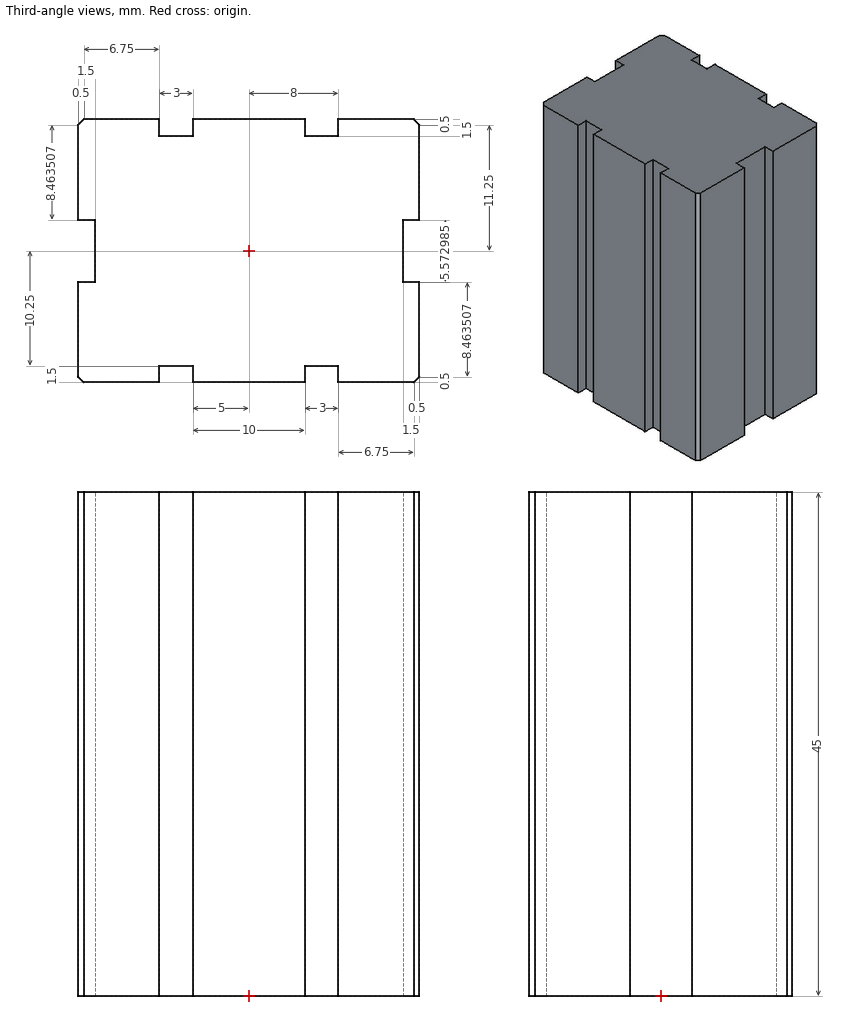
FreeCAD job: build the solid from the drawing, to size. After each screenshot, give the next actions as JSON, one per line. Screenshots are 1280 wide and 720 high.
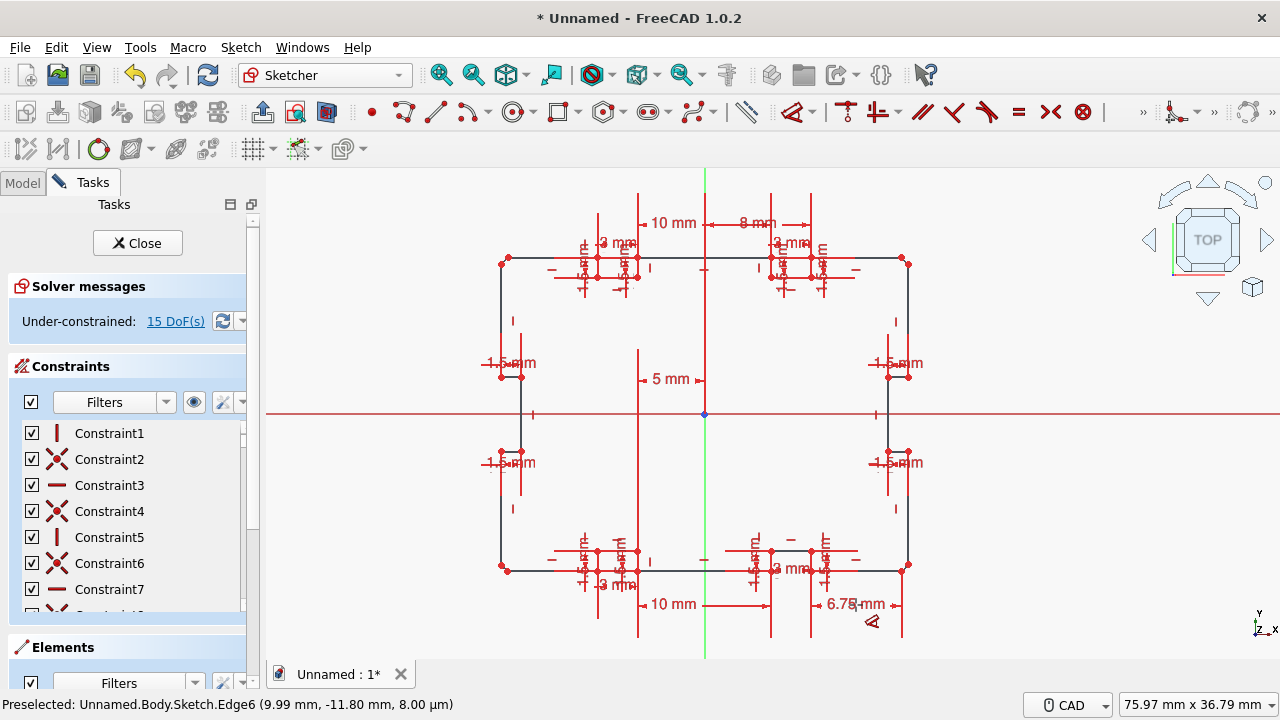
{"action": "left_click", "coordinate": [875, 258]}
{"action": "left_click", "coordinate": [857, 224]}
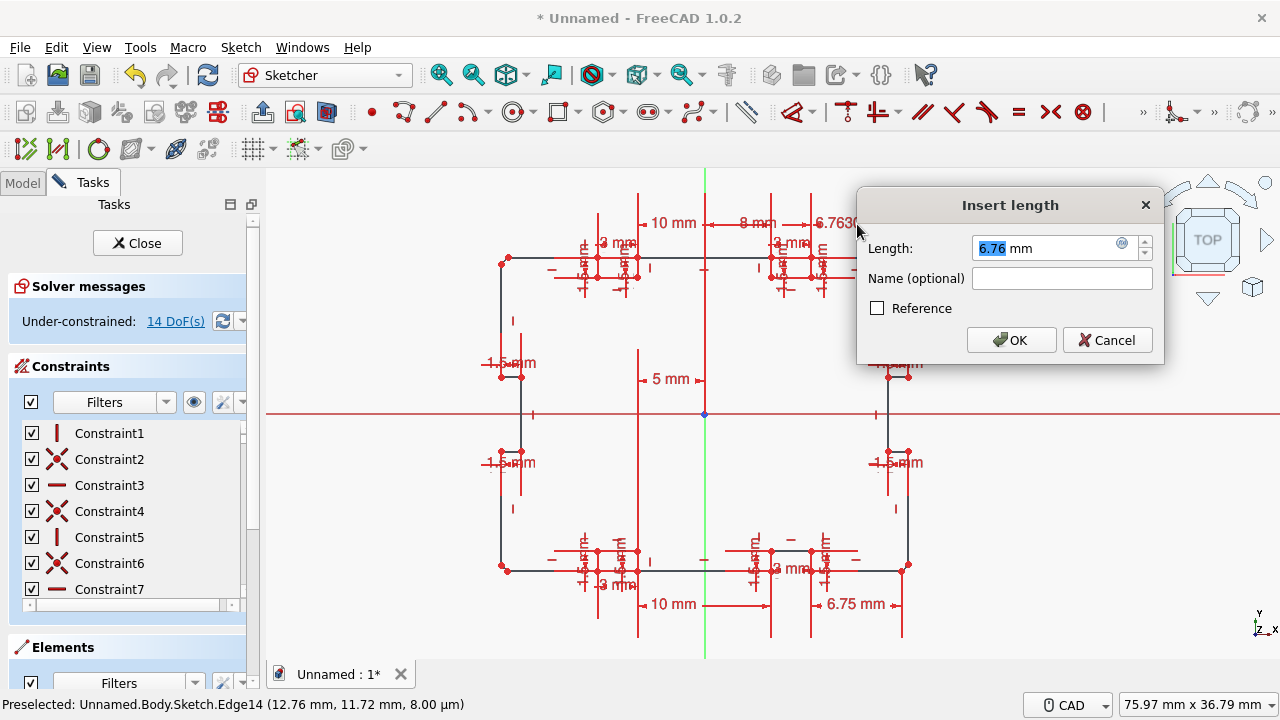
{"action": "type", "text": "6.75"}
{"action": "key", "text": "Return"}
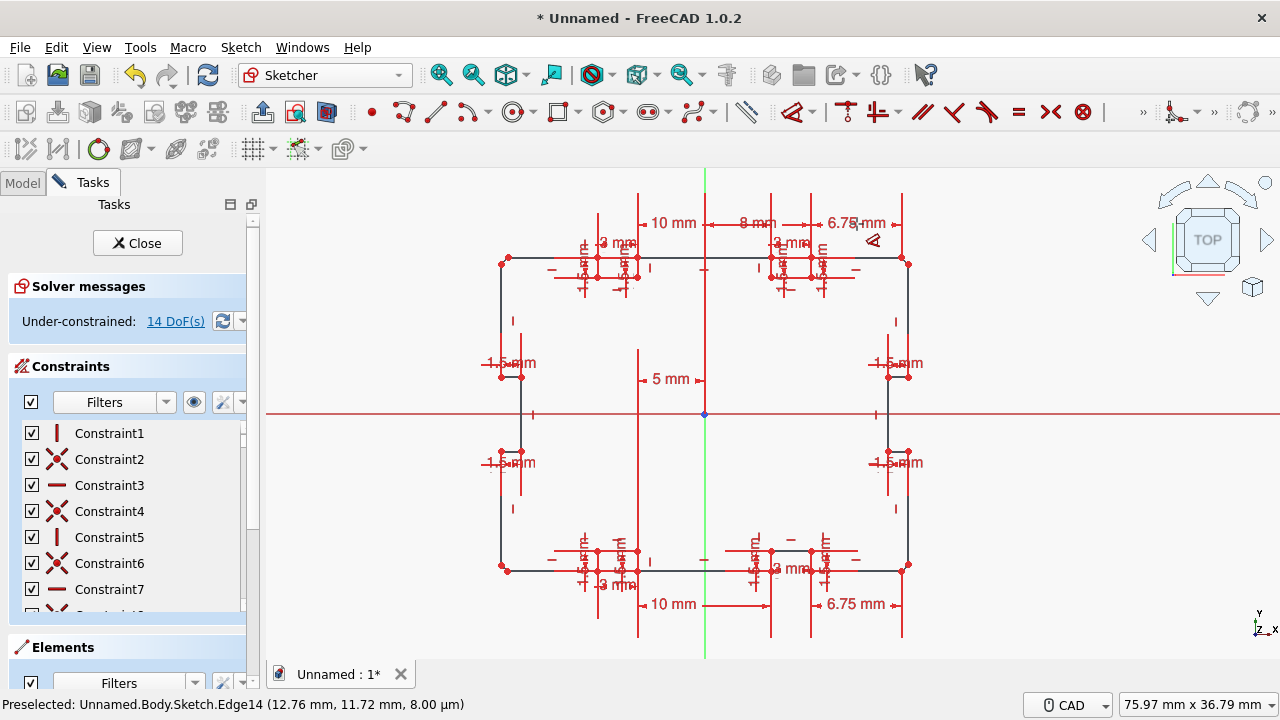
{"action": "left_click", "coordinate": [571, 258]}
{"action": "left_click", "coordinate": [553, 224]}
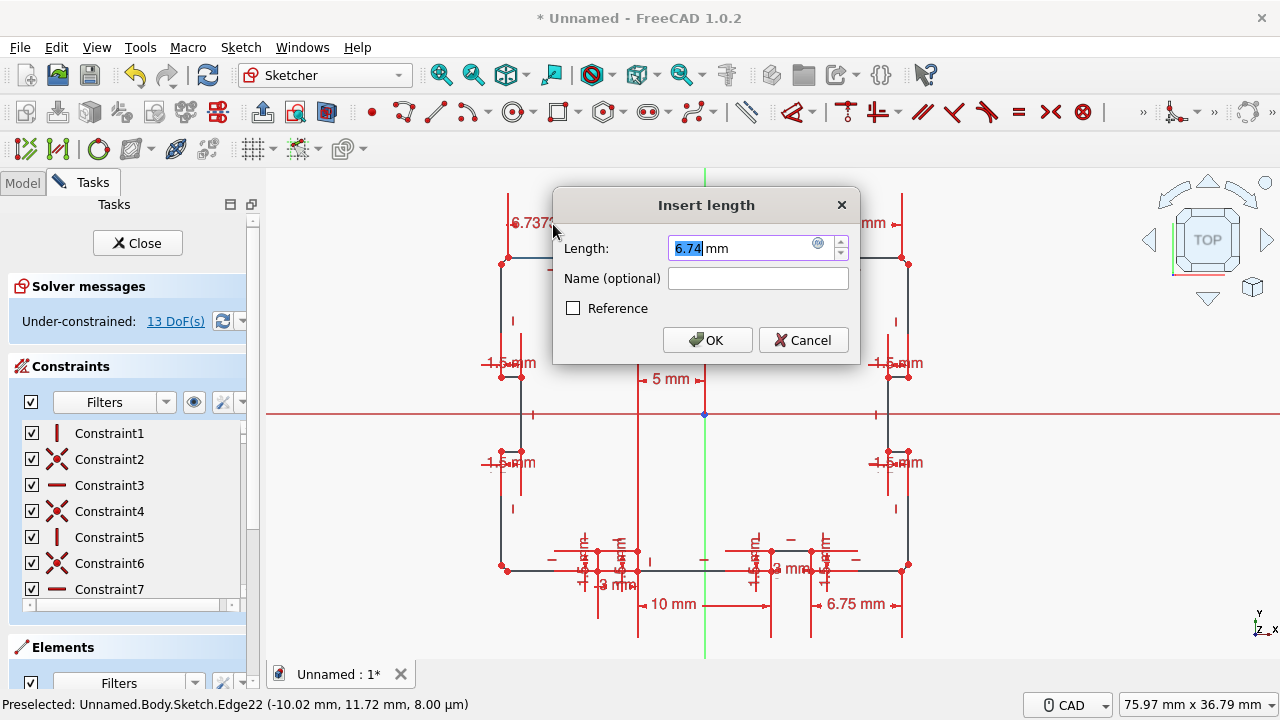
{"action": "type", "text": "6.75"}
{"action": "key", "text": "Return"}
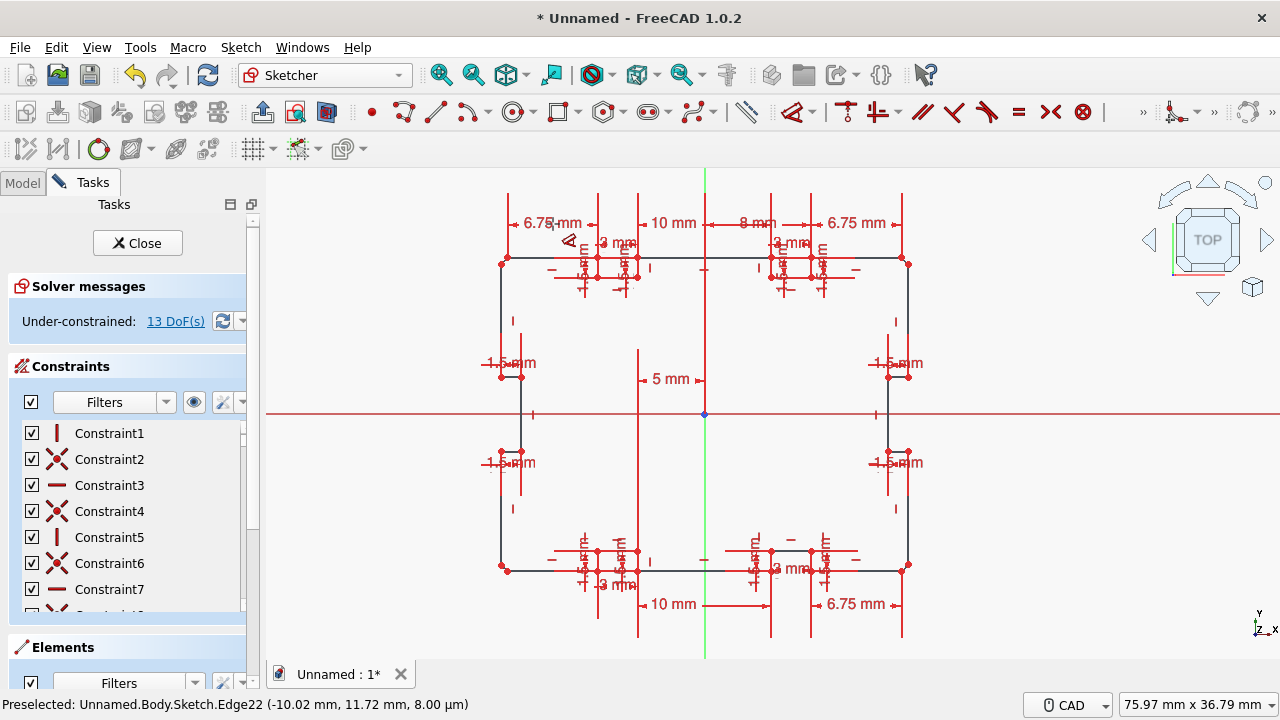
{"action": "left_click", "coordinate": [535, 571]}
{"action": "left_click", "coordinate": [532, 605]}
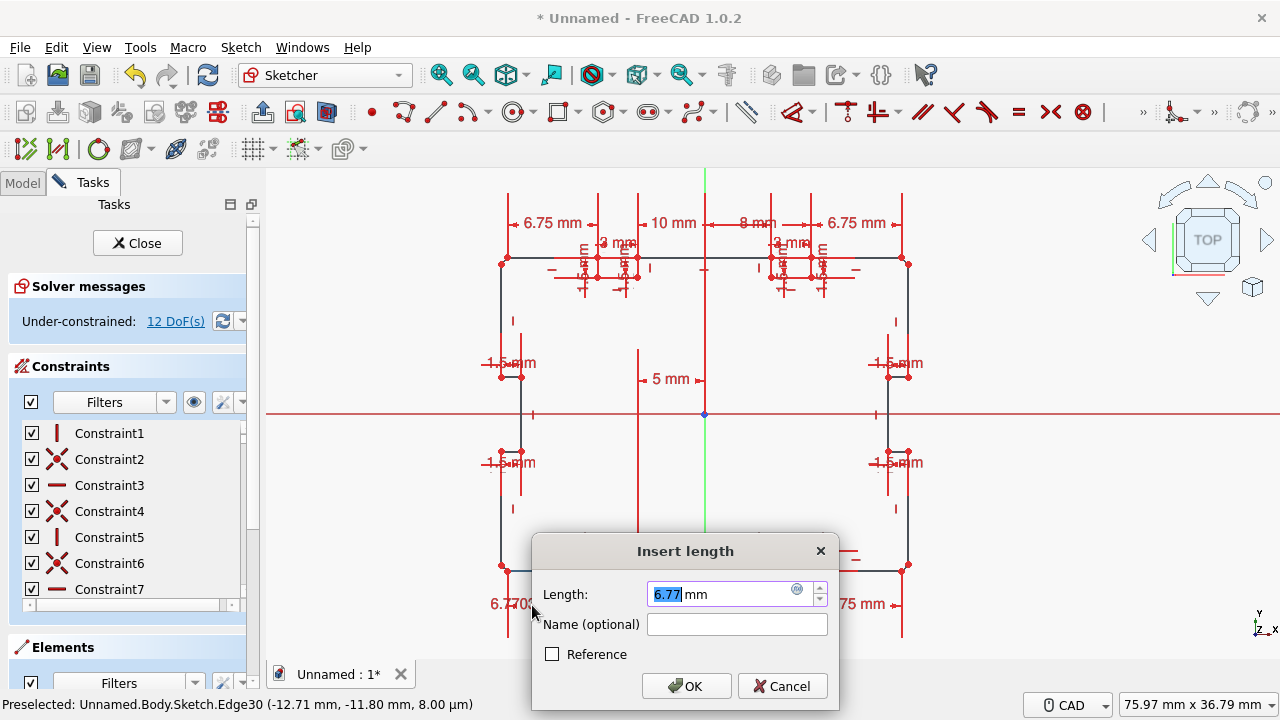
{"action": "type", "text": "6.75"}
{"action": "key", "text": "Return"}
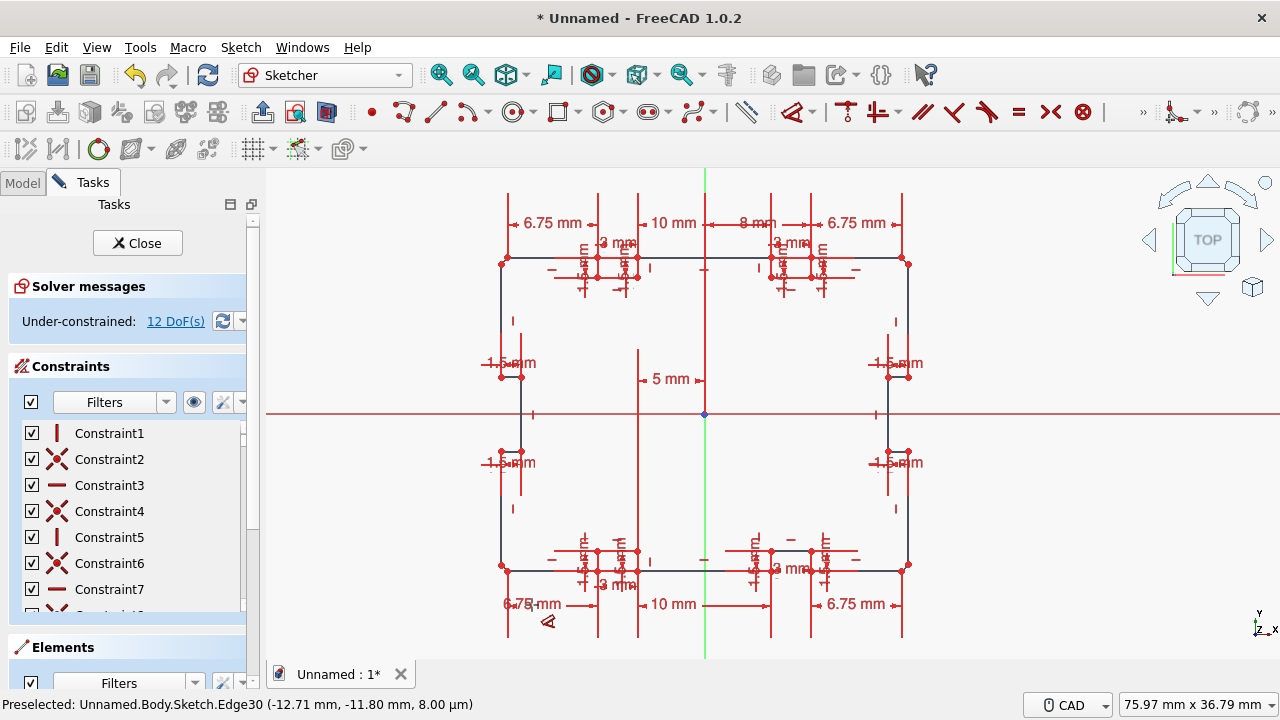
{"action": "scroll", "coordinate": [905, 568], "scroll_direction": "up", "scroll_amount": 9}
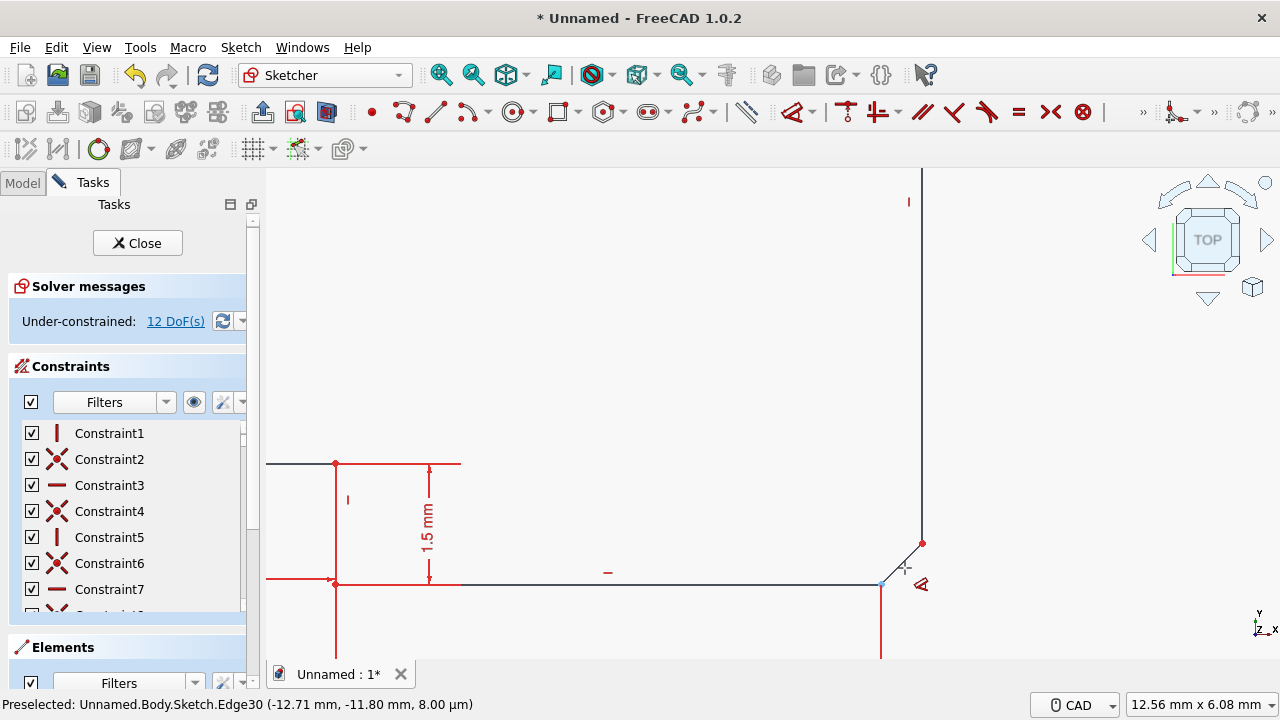
{"action": "left_click", "coordinate": [902, 564]}
{"action": "left_click", "coordinate": [902, 619]}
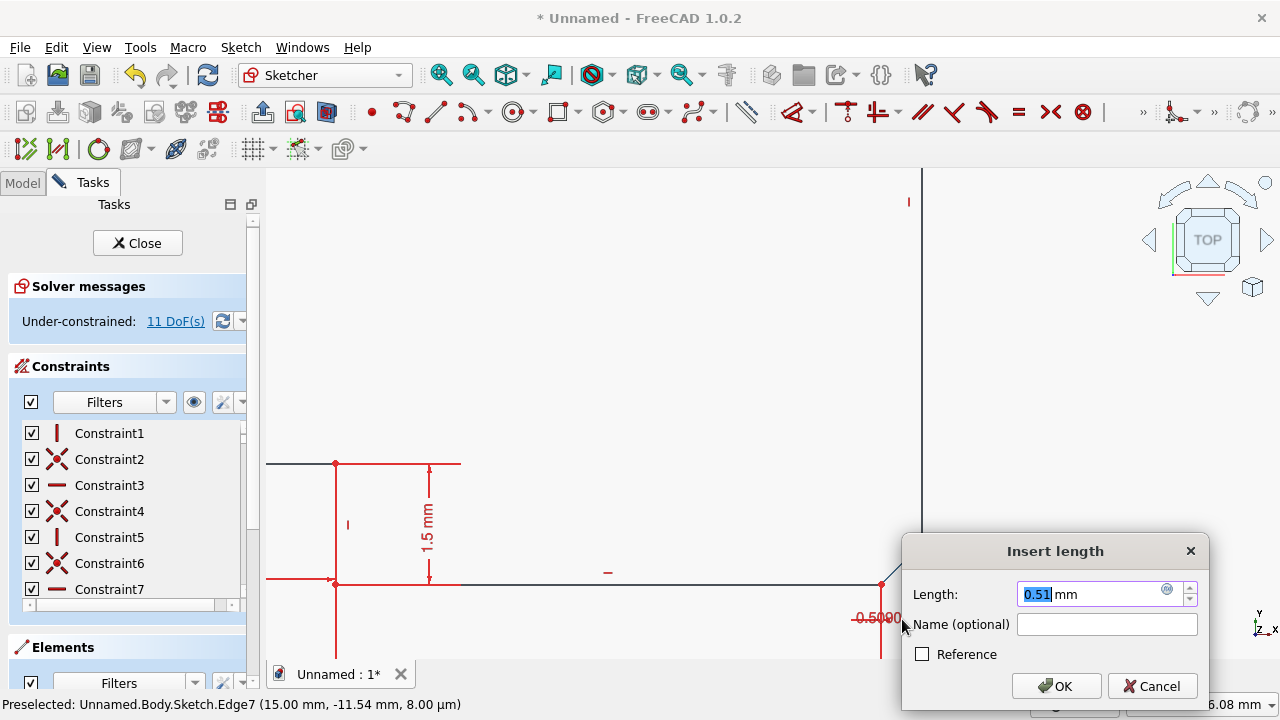
{"action": "type", "text": "0.5"}
{"action": "key", "text": "Return"}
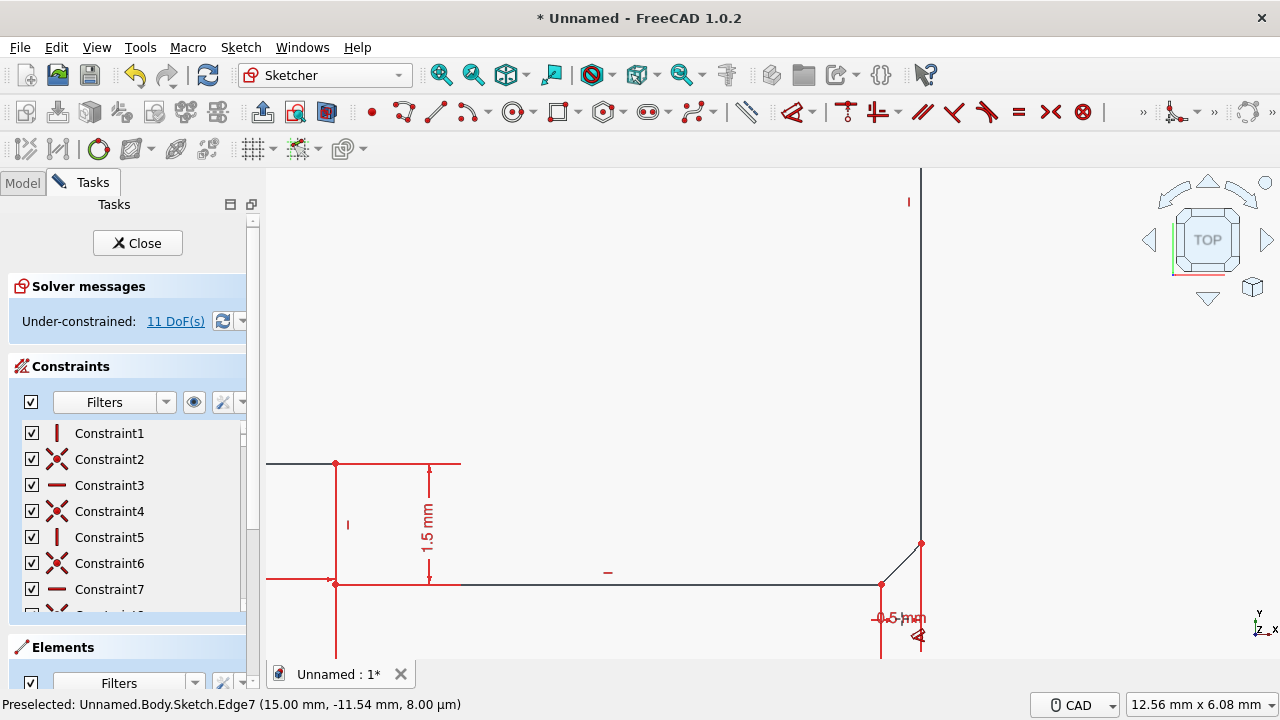
{"action": "left_click", "coordinate": [893, 572]}
{"action": "left_click", "coordinate": [955, 564]}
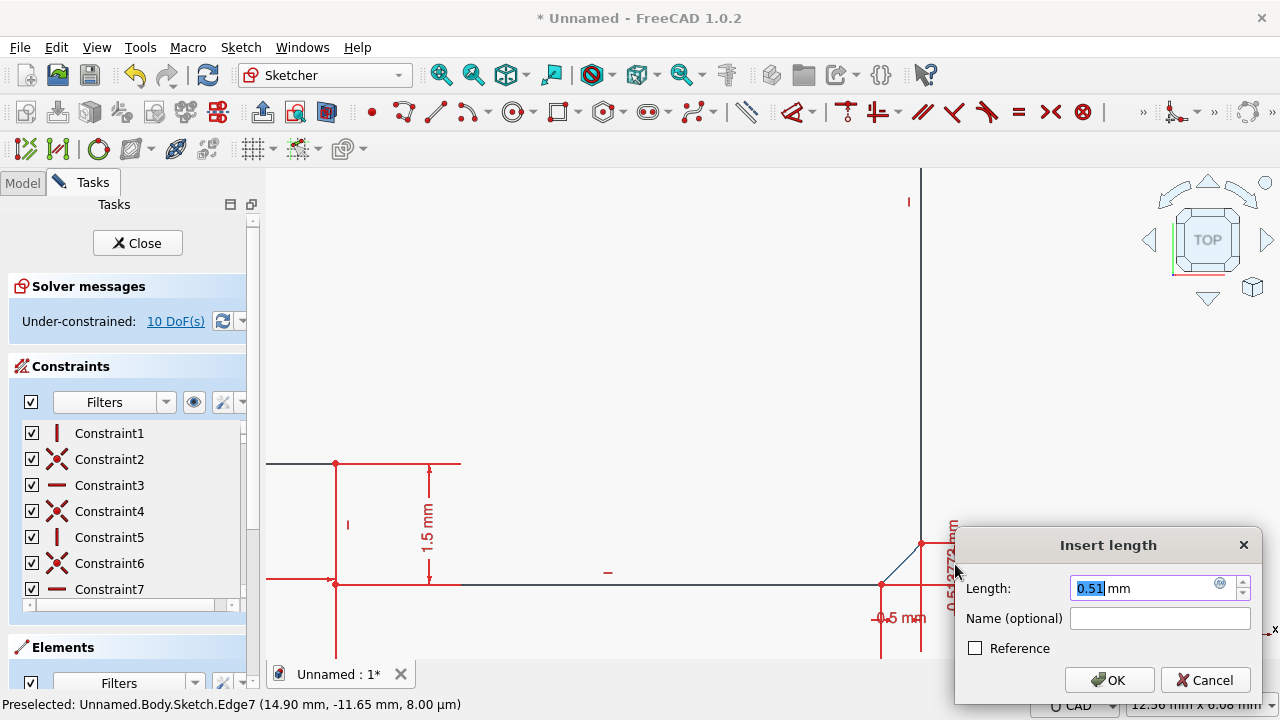
{"action": "type", "text": "0.5"}
{"action": "key", "text": "Return"}